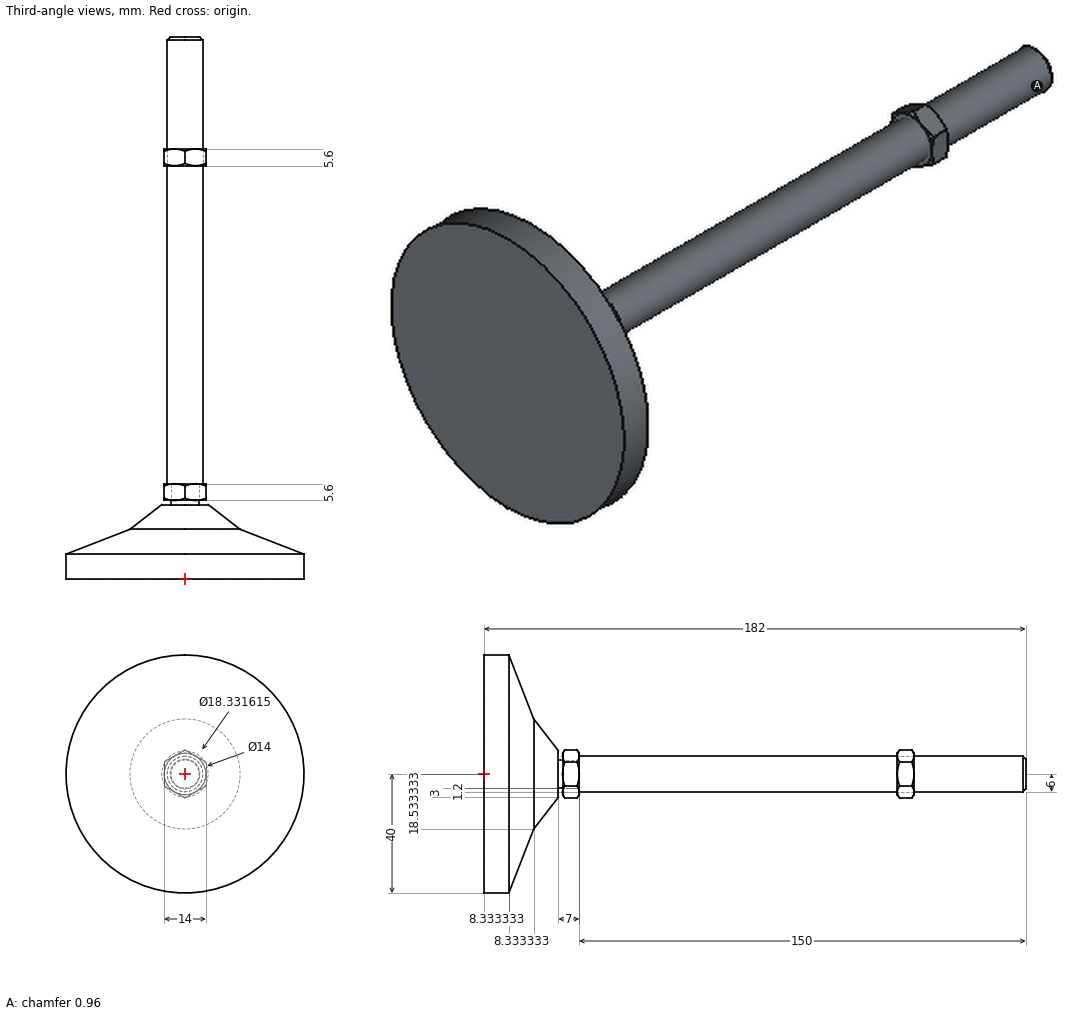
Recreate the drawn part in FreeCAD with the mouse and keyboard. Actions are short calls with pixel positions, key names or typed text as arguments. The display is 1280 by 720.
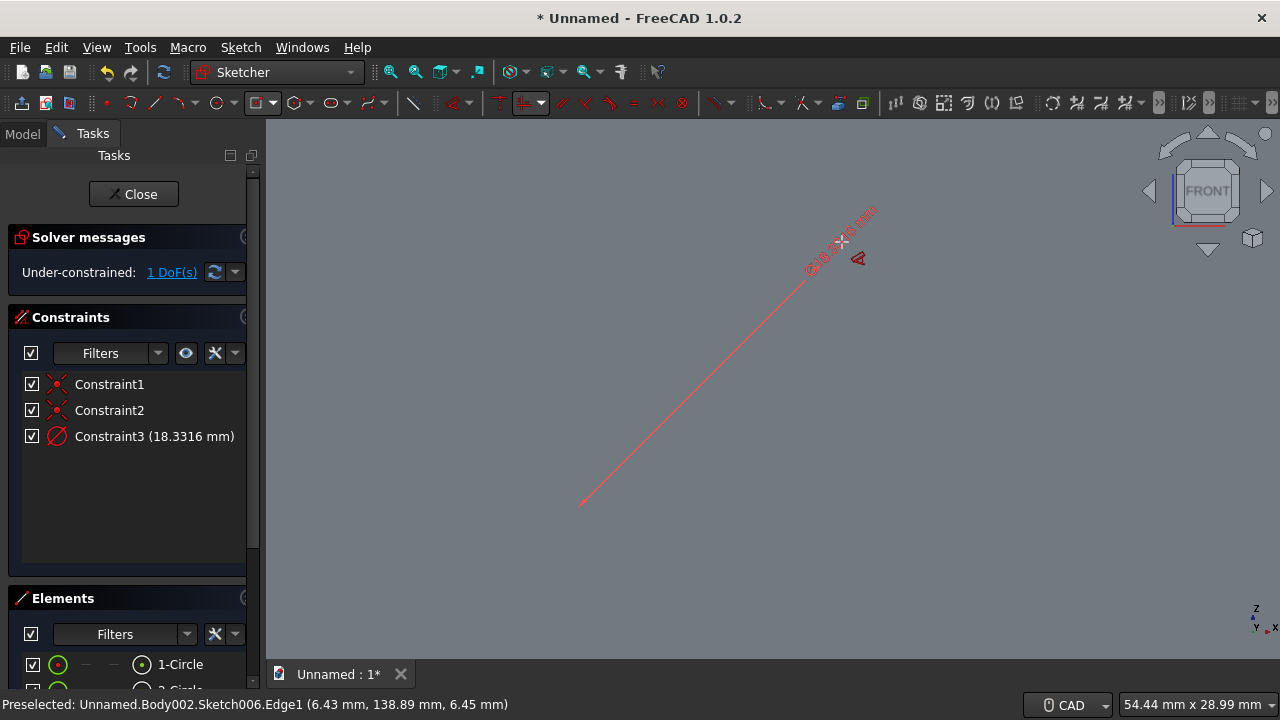
click(791, 294)
click(877, 334)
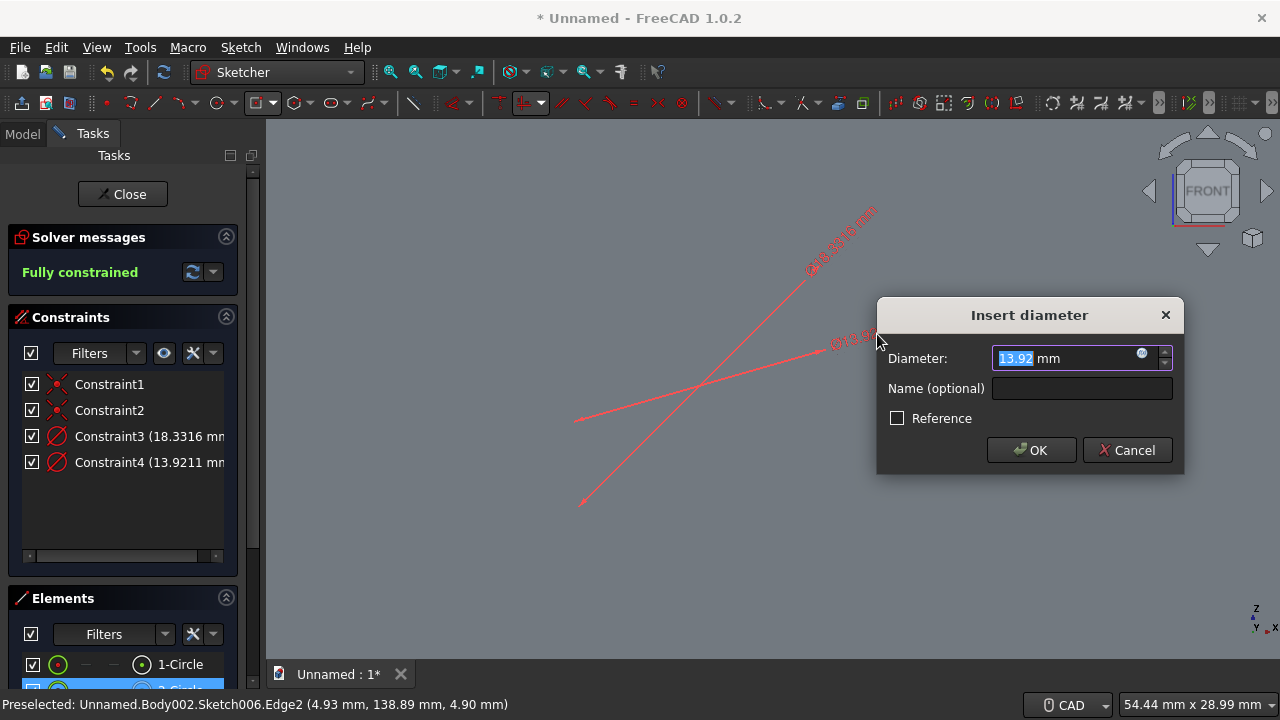
text(14)
key(Return)
key(Escape)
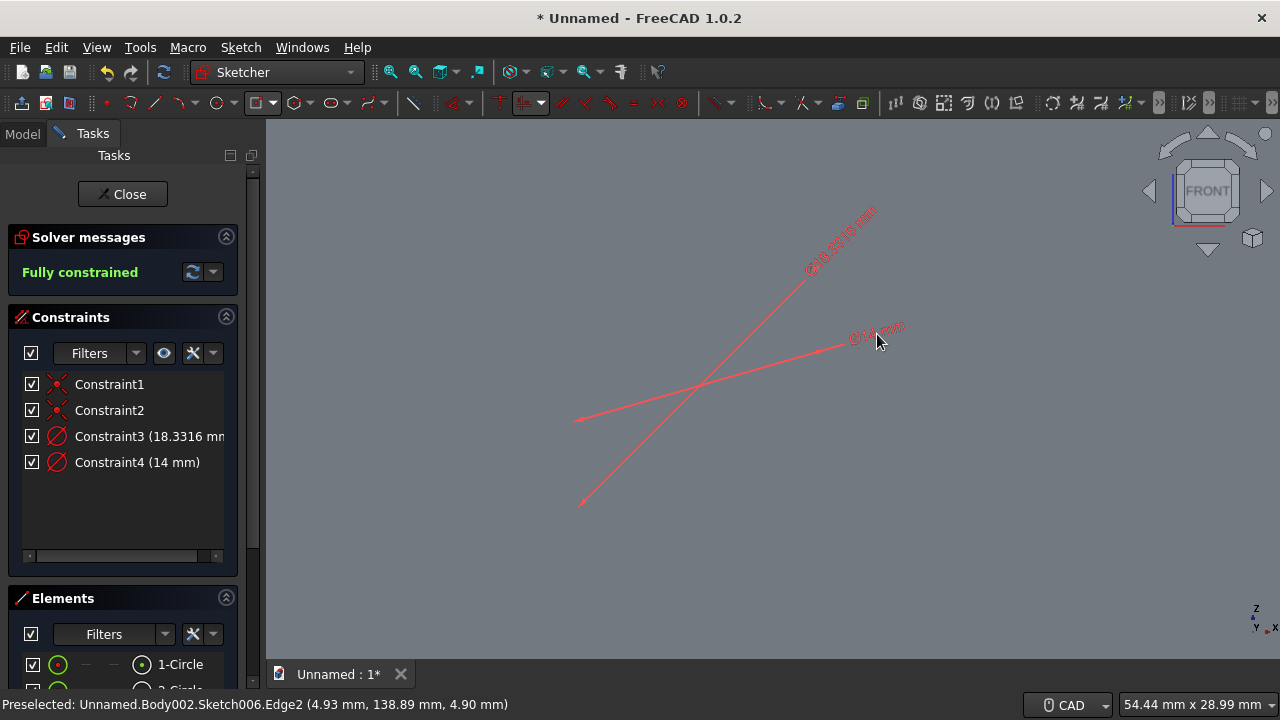
click(123, 194)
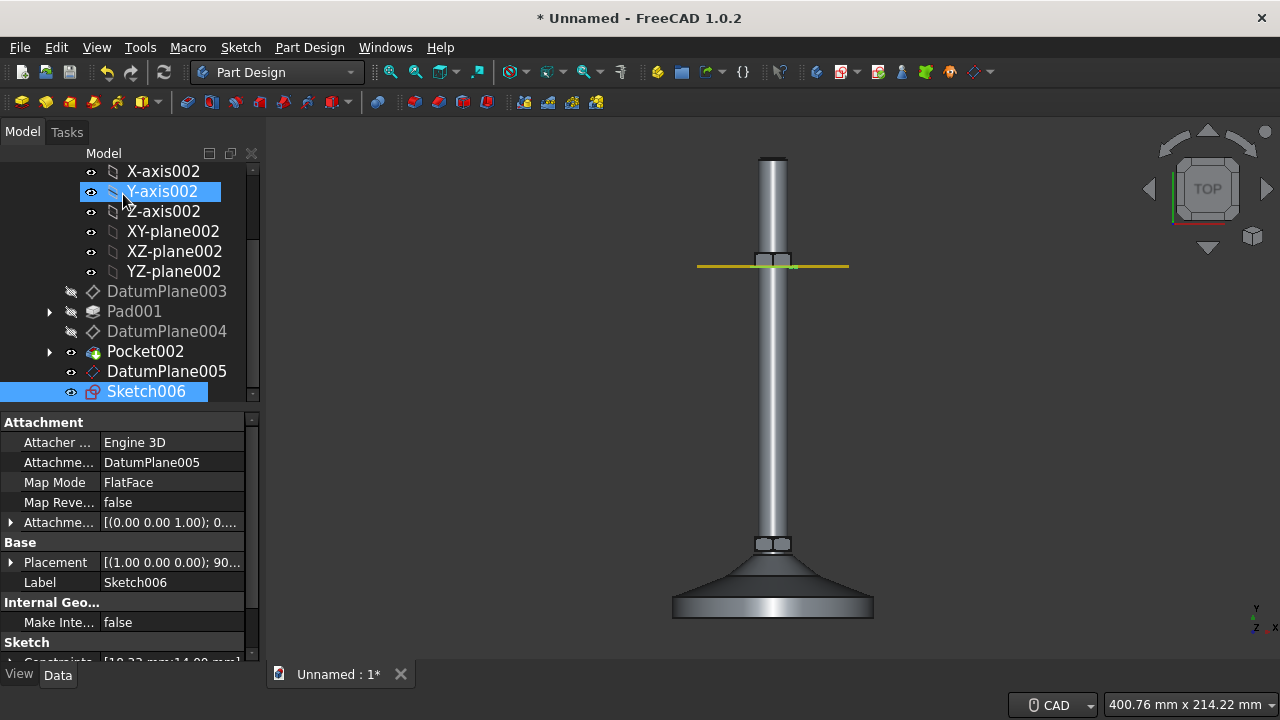
click(188, 102)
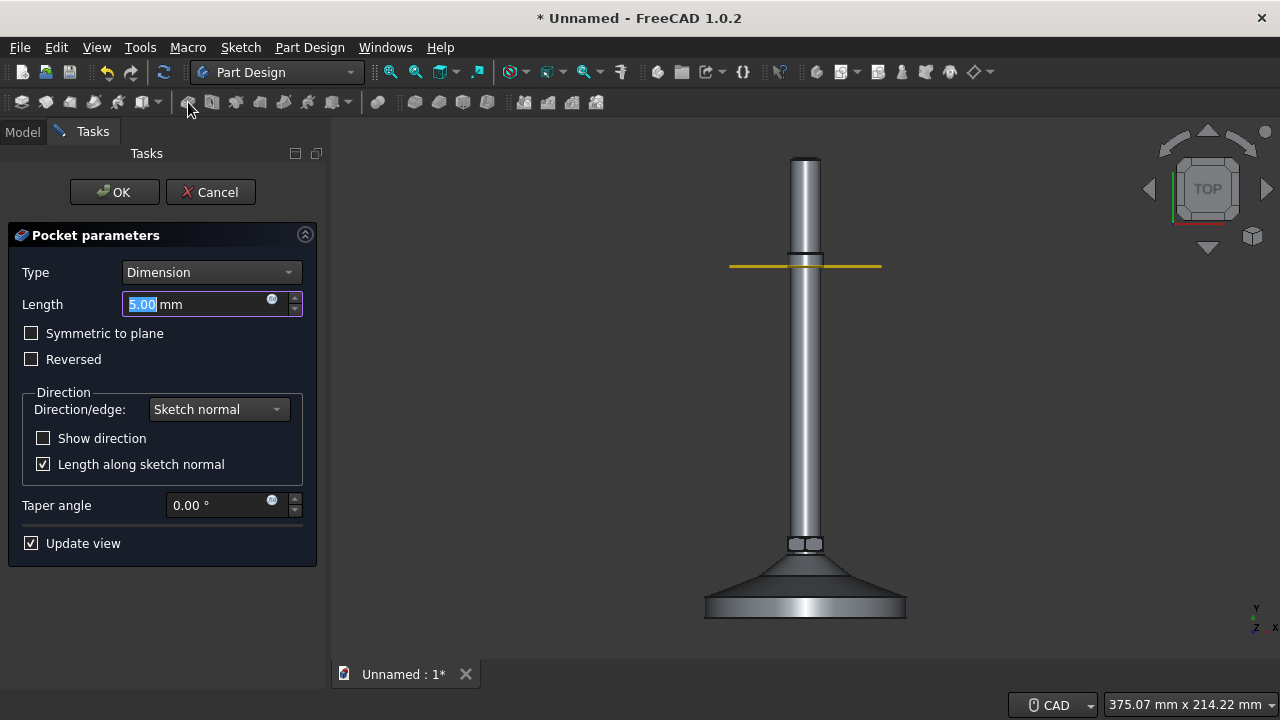
text(5.6)
key(Tab)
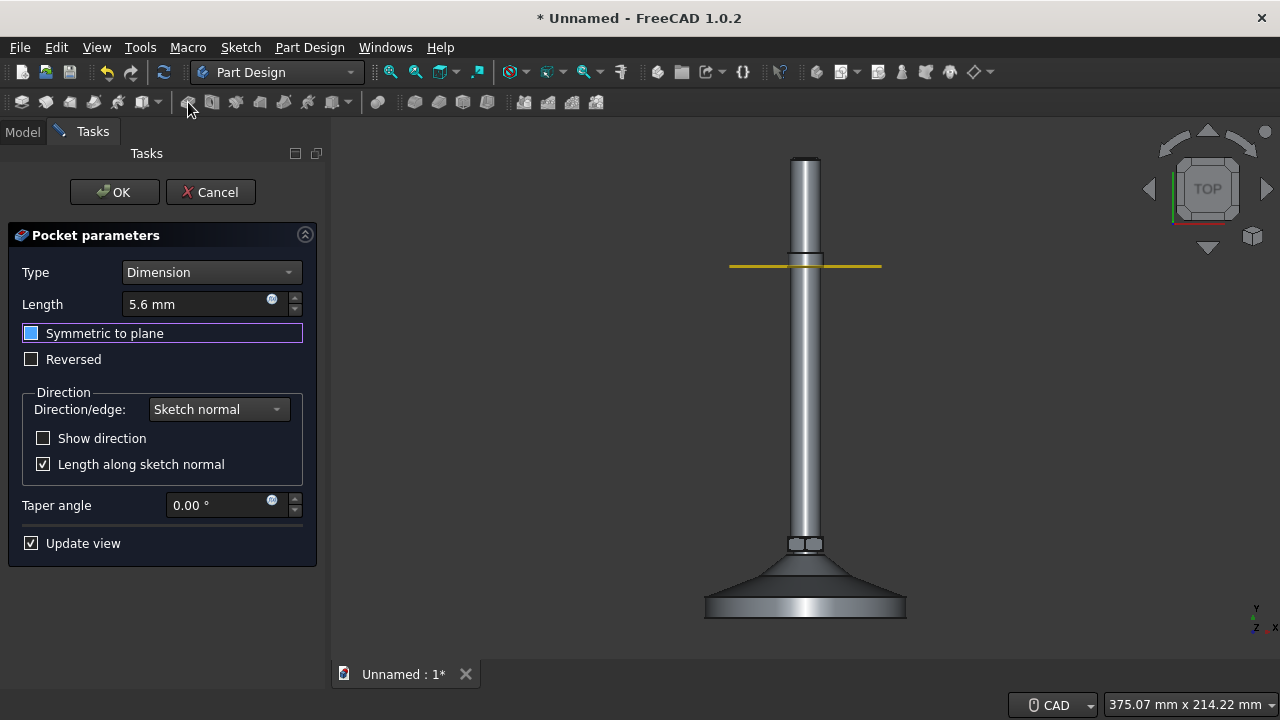
triple_click(226, 505)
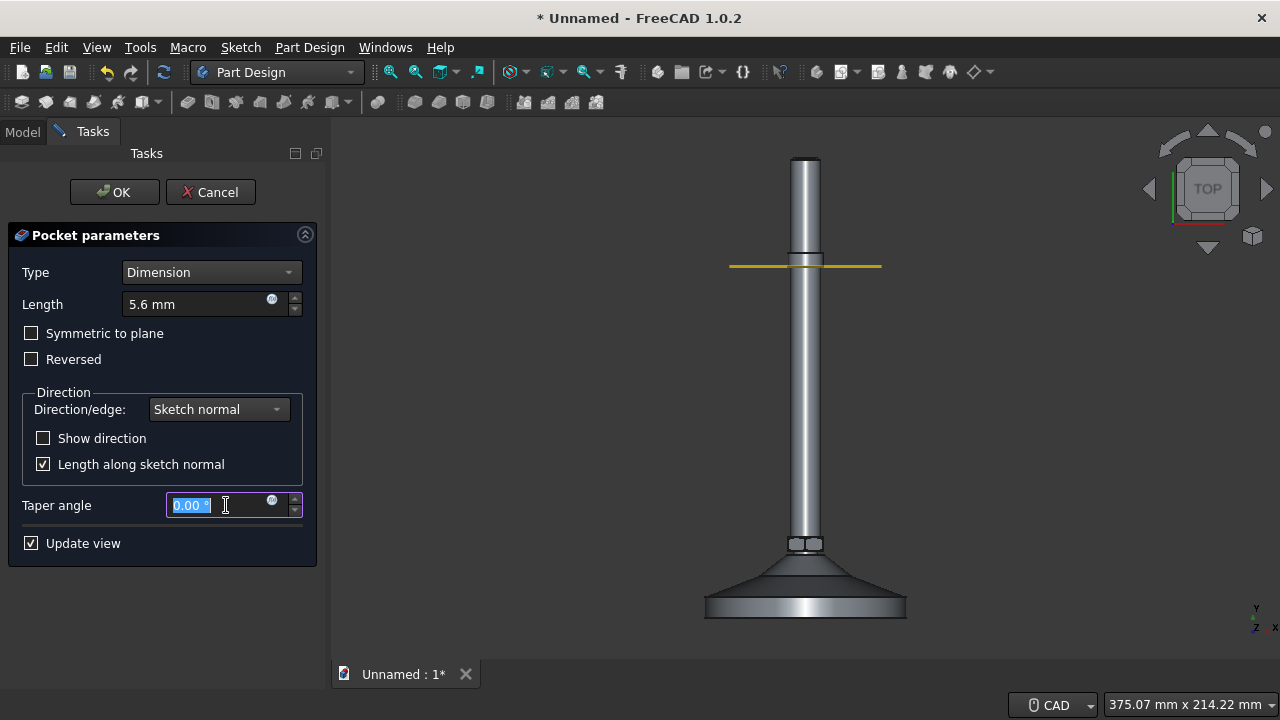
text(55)
key(Tab)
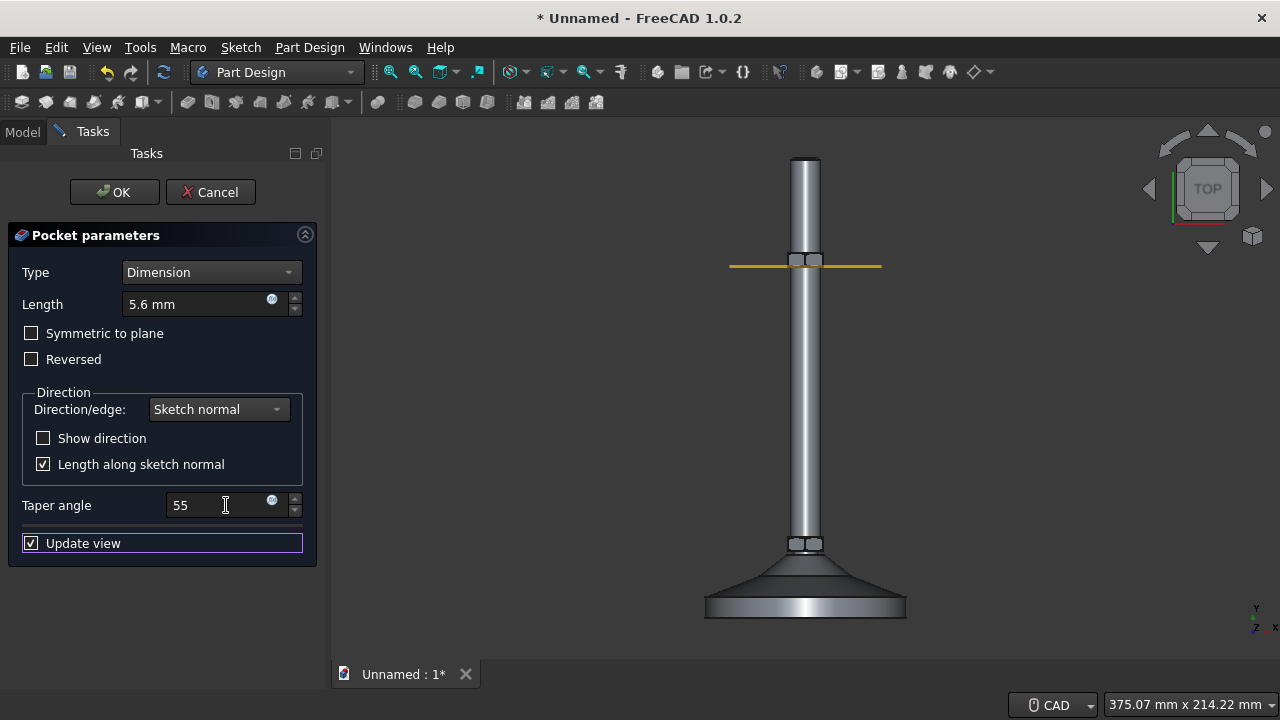
click(115, 192)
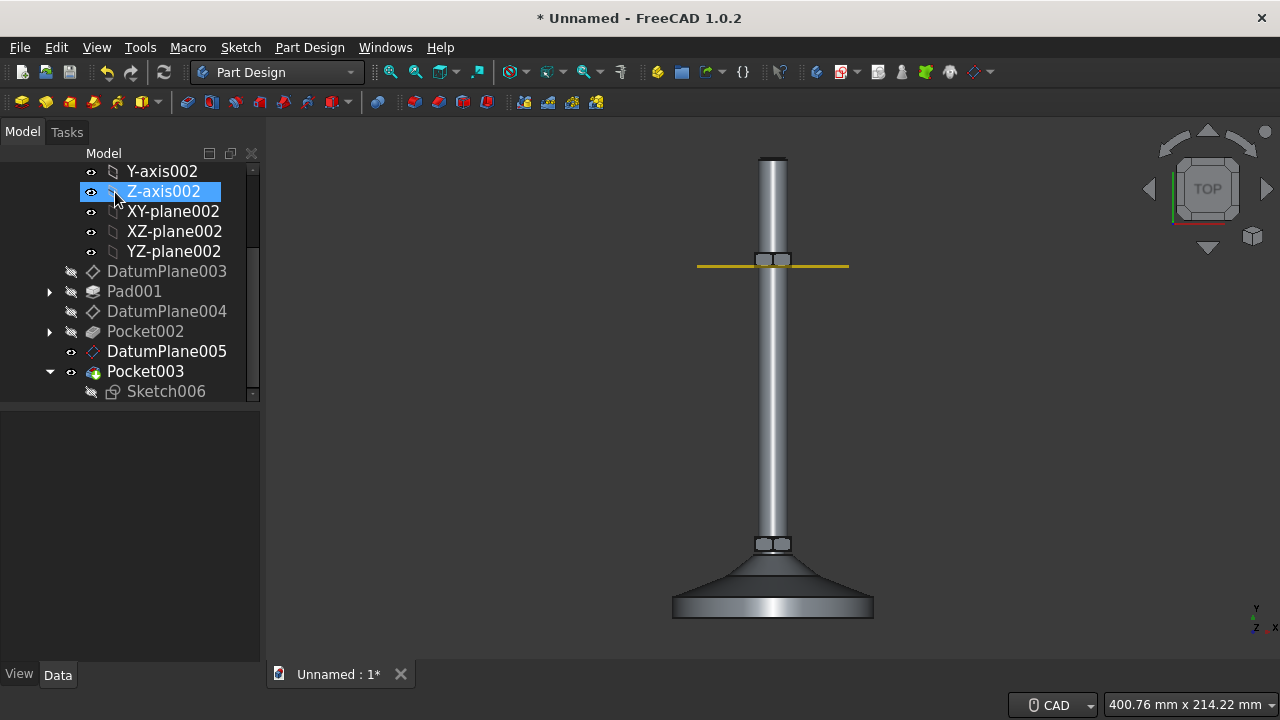
click(116, 352)
key(space)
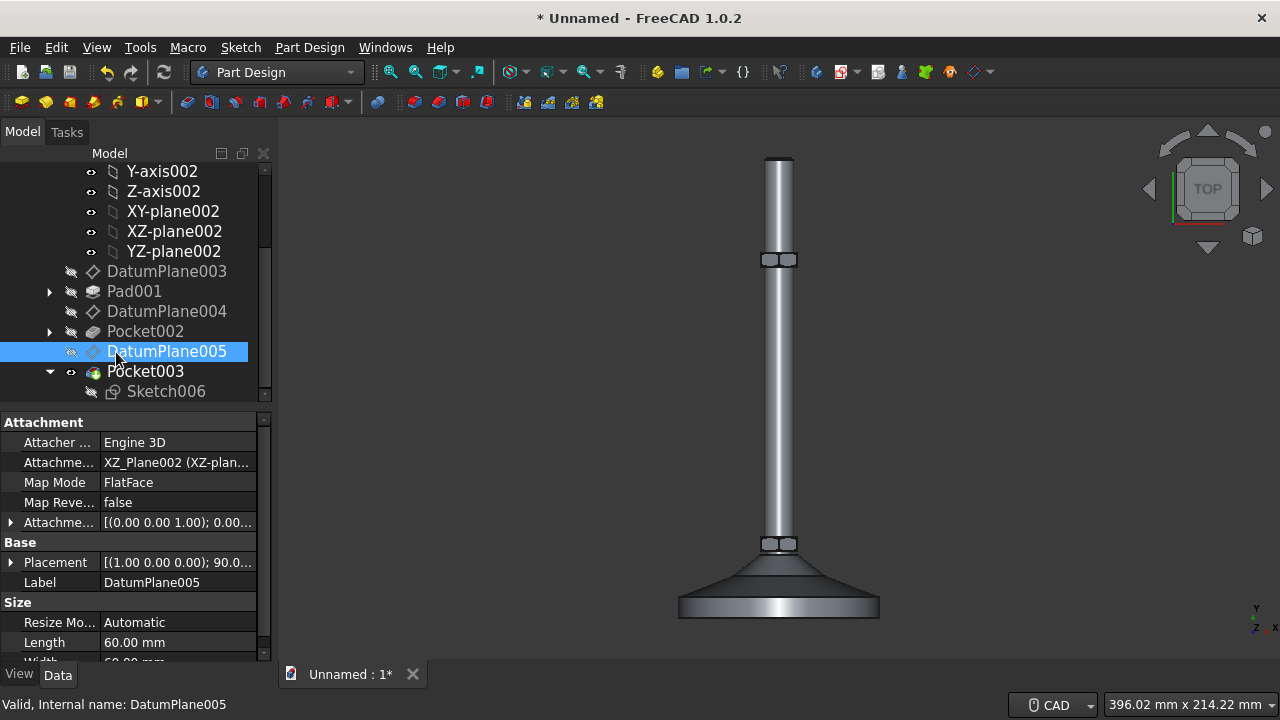
key(0)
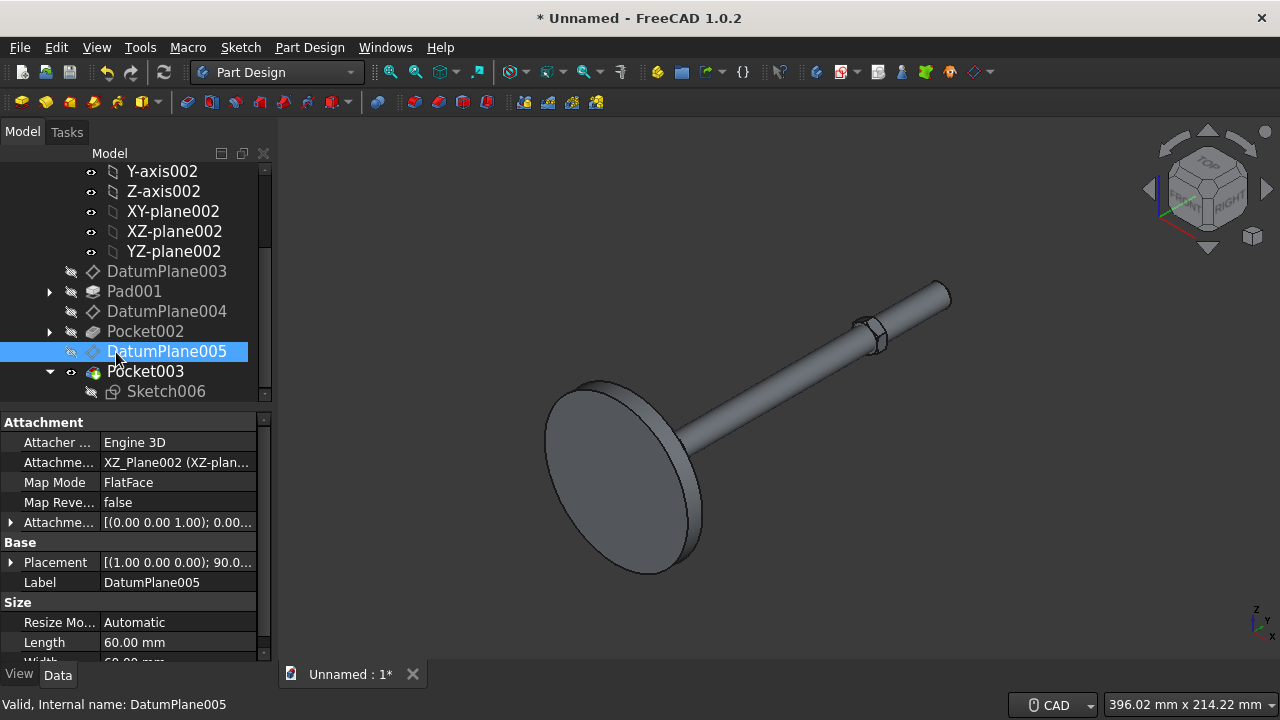
click(392, 72)